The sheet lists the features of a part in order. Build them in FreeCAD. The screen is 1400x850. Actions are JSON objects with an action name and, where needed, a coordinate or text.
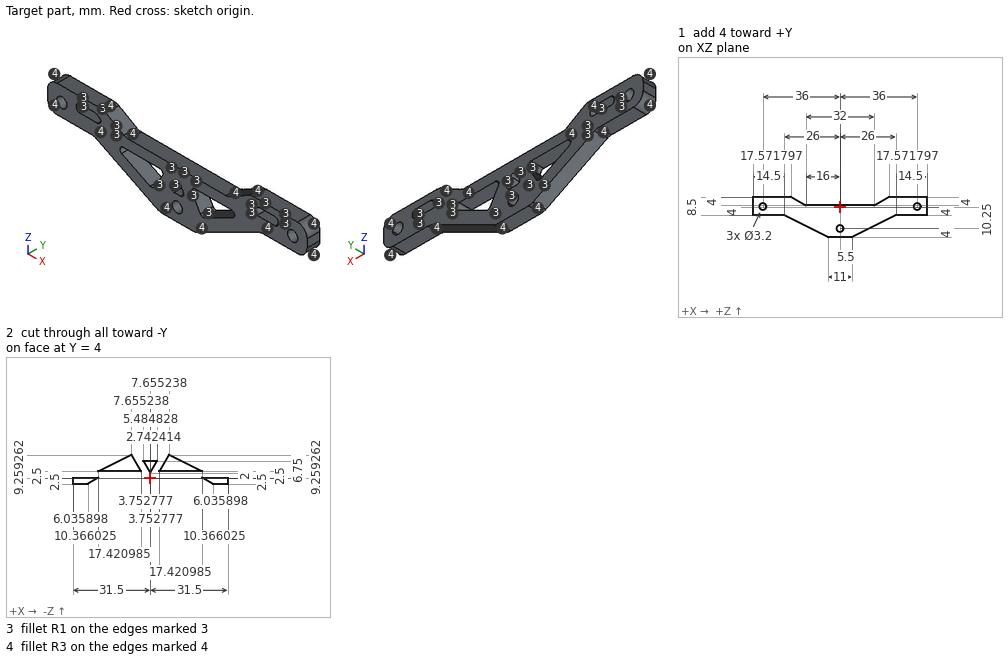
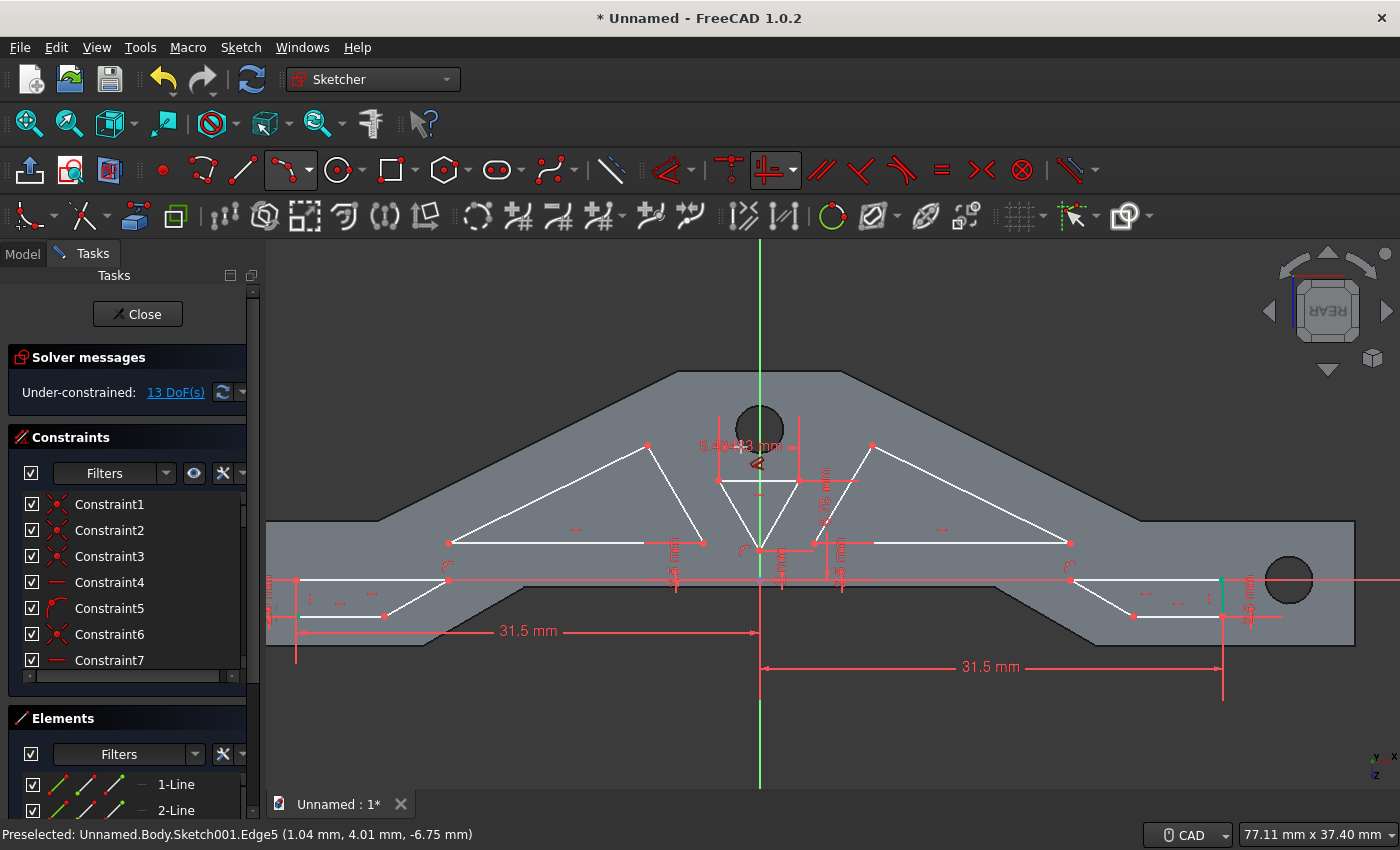
{"action": "left_click", "coordinate": [323, 617]}
{"action": "left_click", "coordinate": [341, 651]}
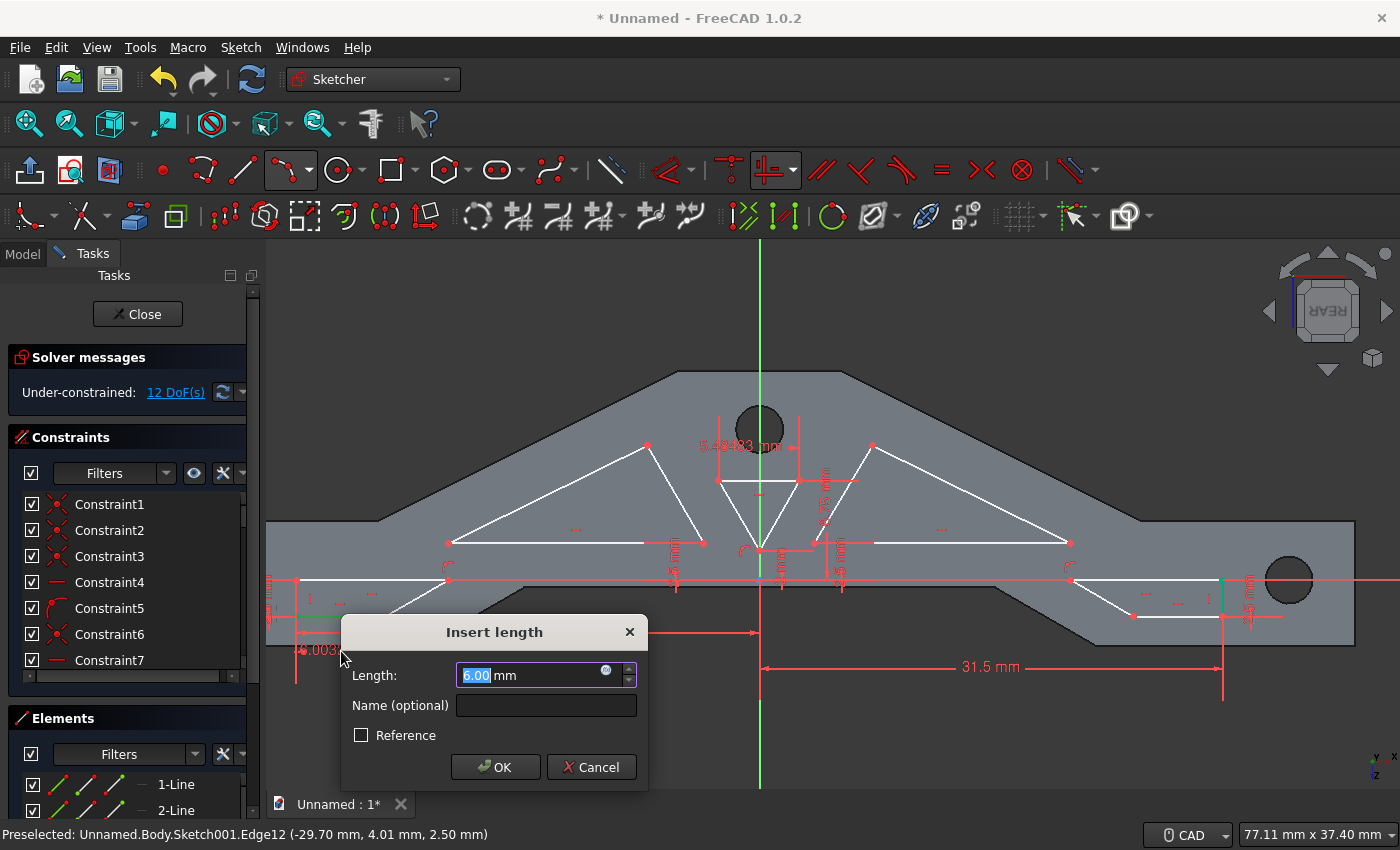
{"action": "type", "text": "6.035898"}
{"action": "key", "text": "Return"}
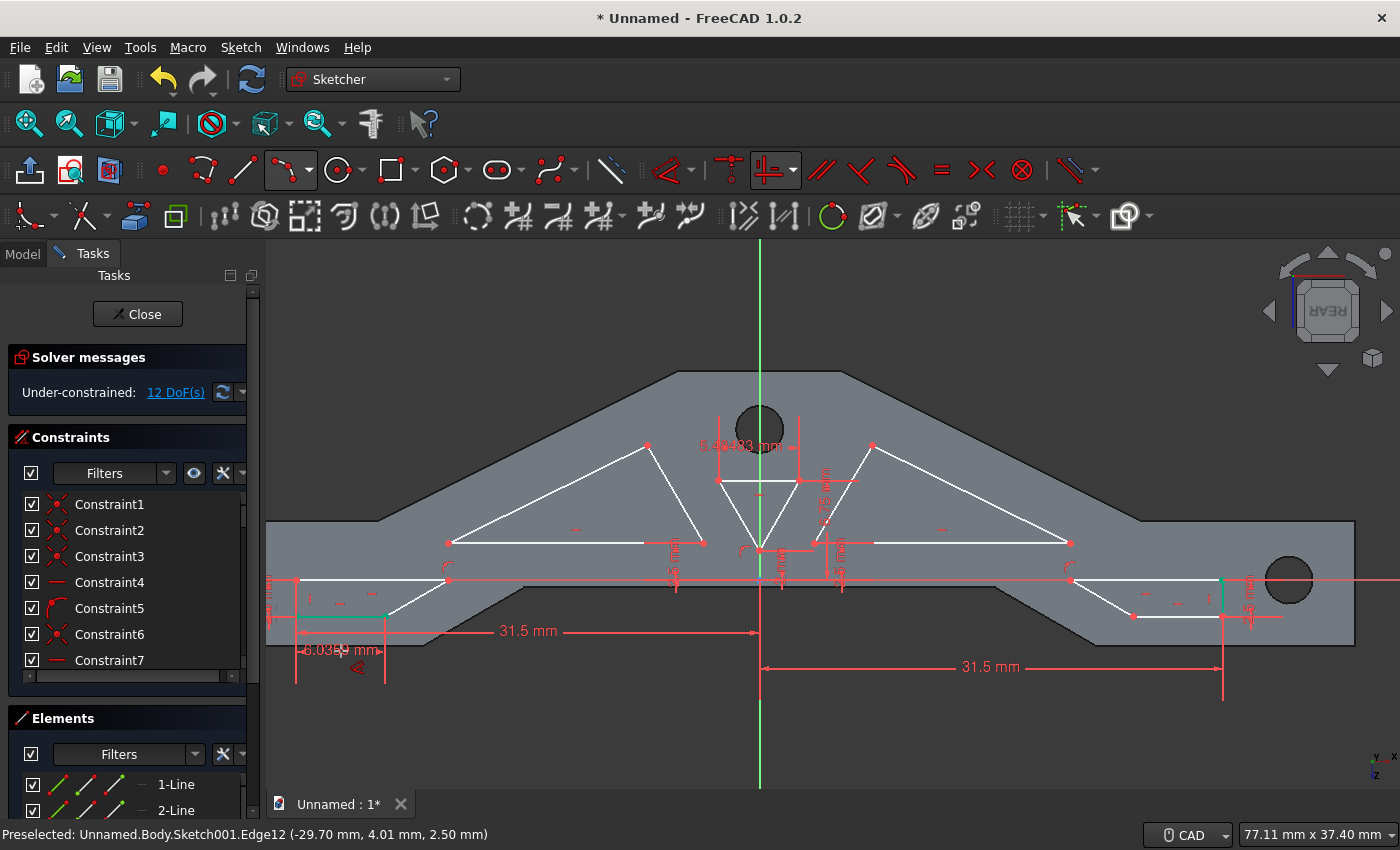
{"action": "left_click", "coordinate": [1160, 617]}
{"action": "left_click", "coordinate": [1178, 651]}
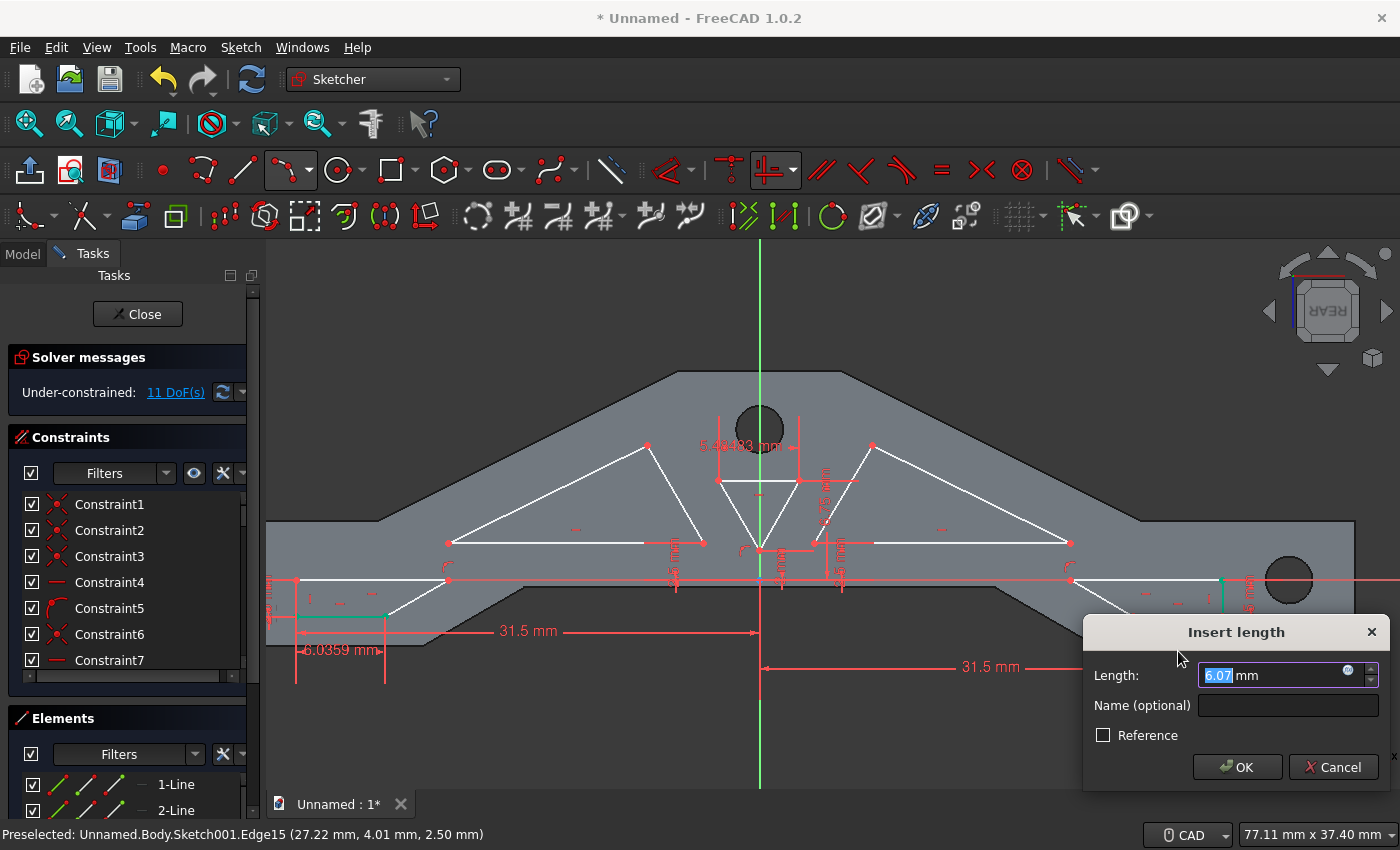
{"action": "type", "text": "6.035898"}
{"action": "key", "text": "Return"}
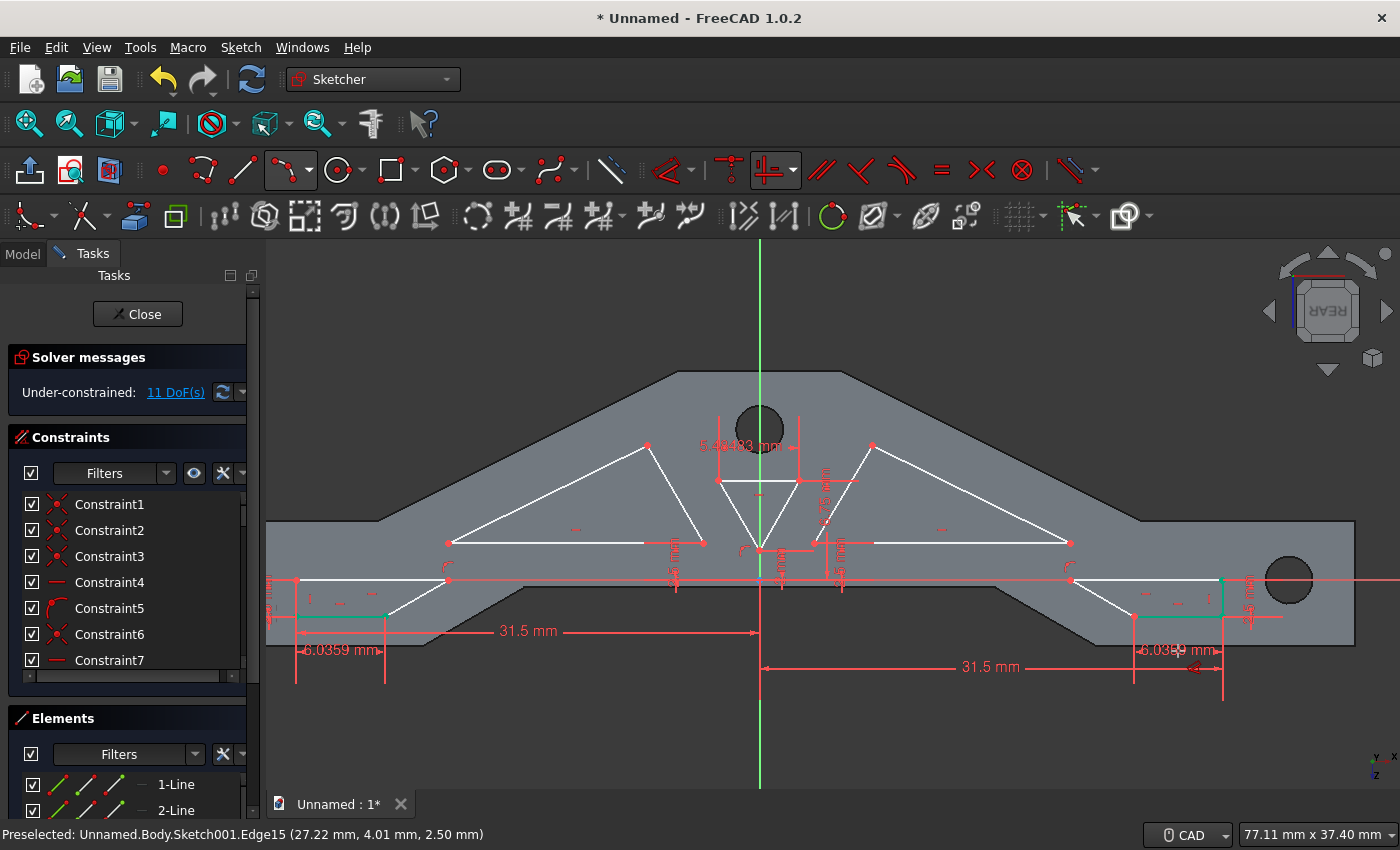
{"action": "left_click", "coordinate": [525, 543]}
{"action": "left_click", "coordinate": [576, 509]}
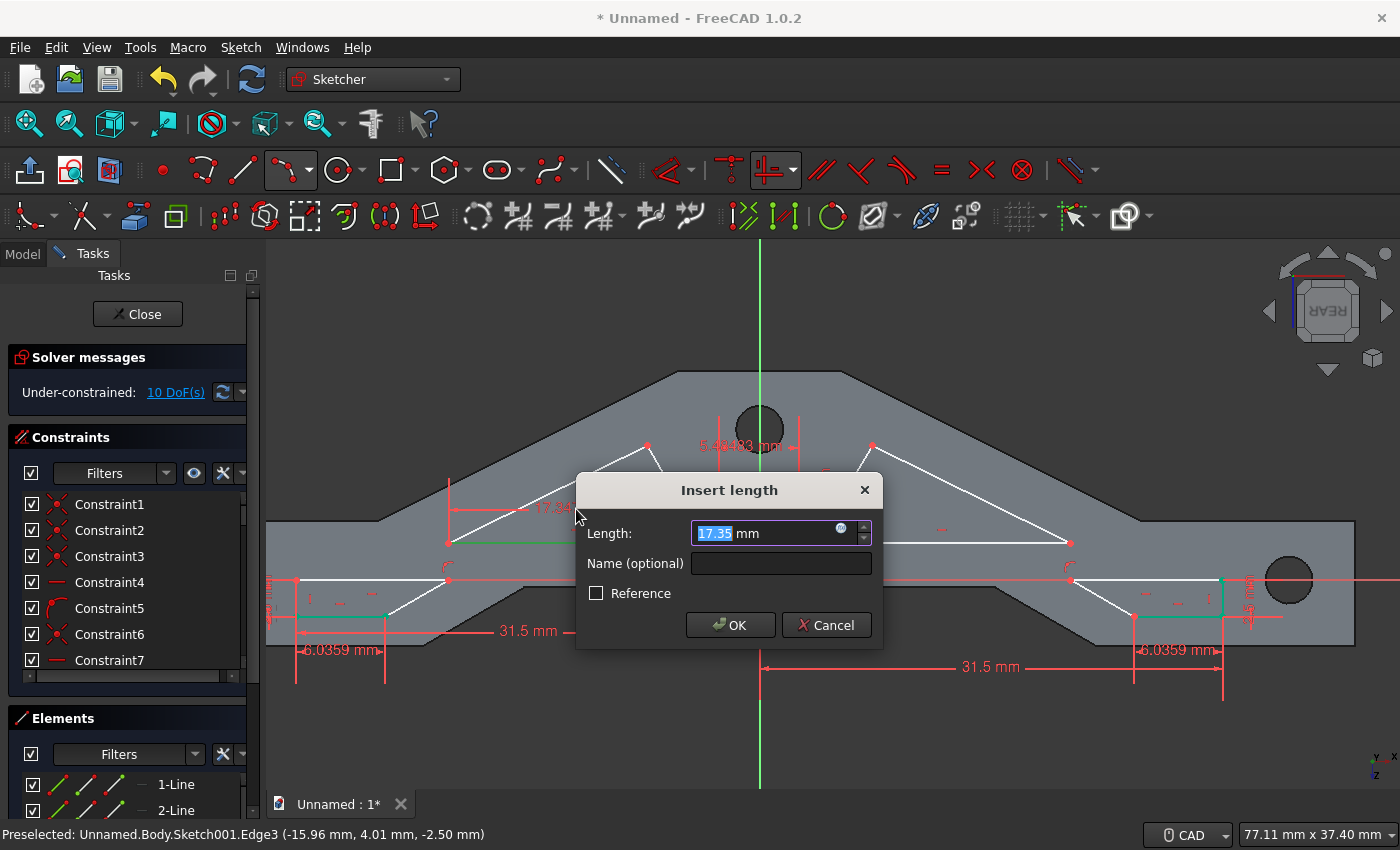
{"action": "type", "text": "17.420985"}
{"action": "key", "text": "Return"}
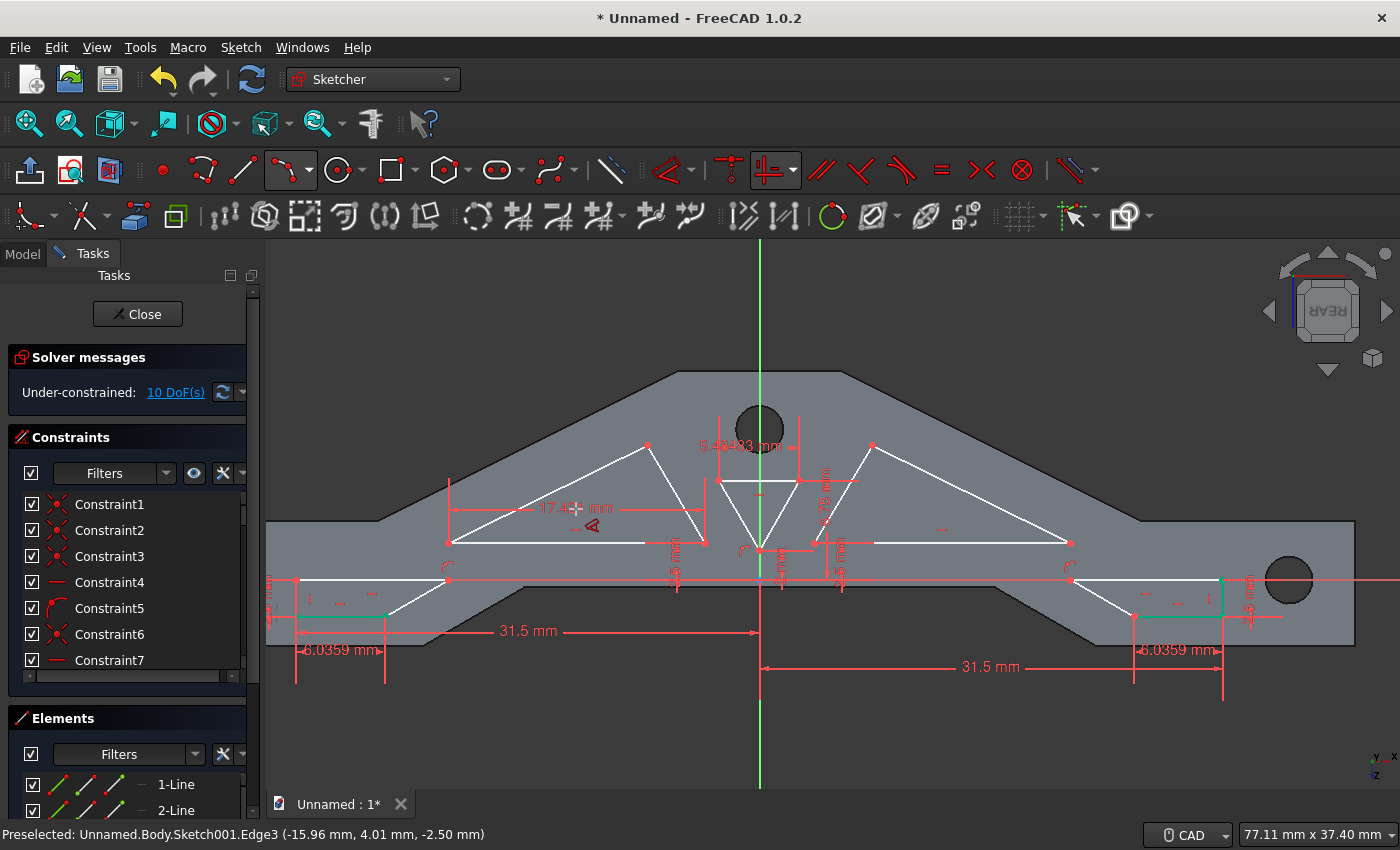
{"action": "left_click", "coordinate": [891, 543]}
{"action": "left_click", "coordinate": [943, 509]}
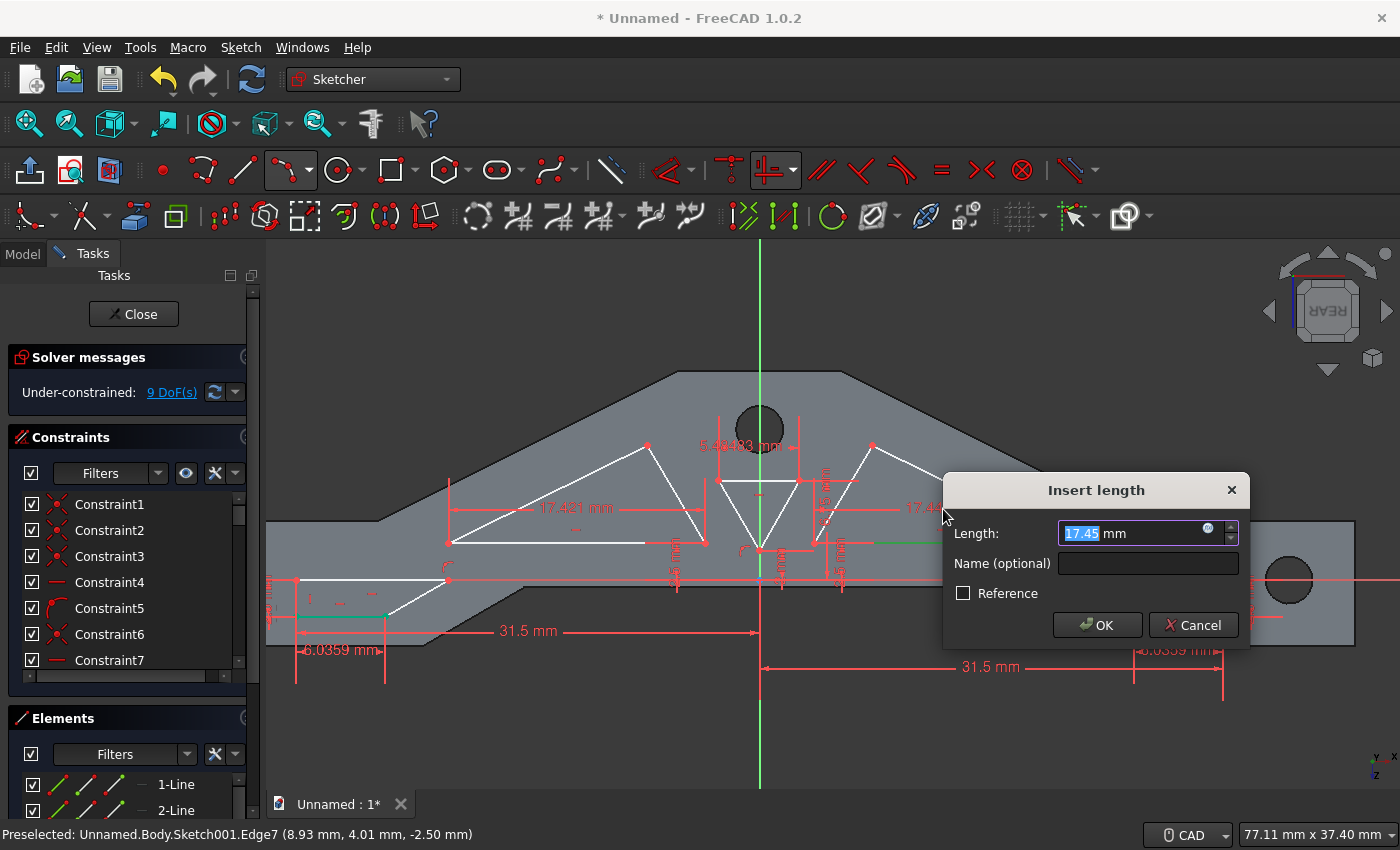
{"action": "type", "text": "17.420985"}
{"action": "key", "text": "Return"}